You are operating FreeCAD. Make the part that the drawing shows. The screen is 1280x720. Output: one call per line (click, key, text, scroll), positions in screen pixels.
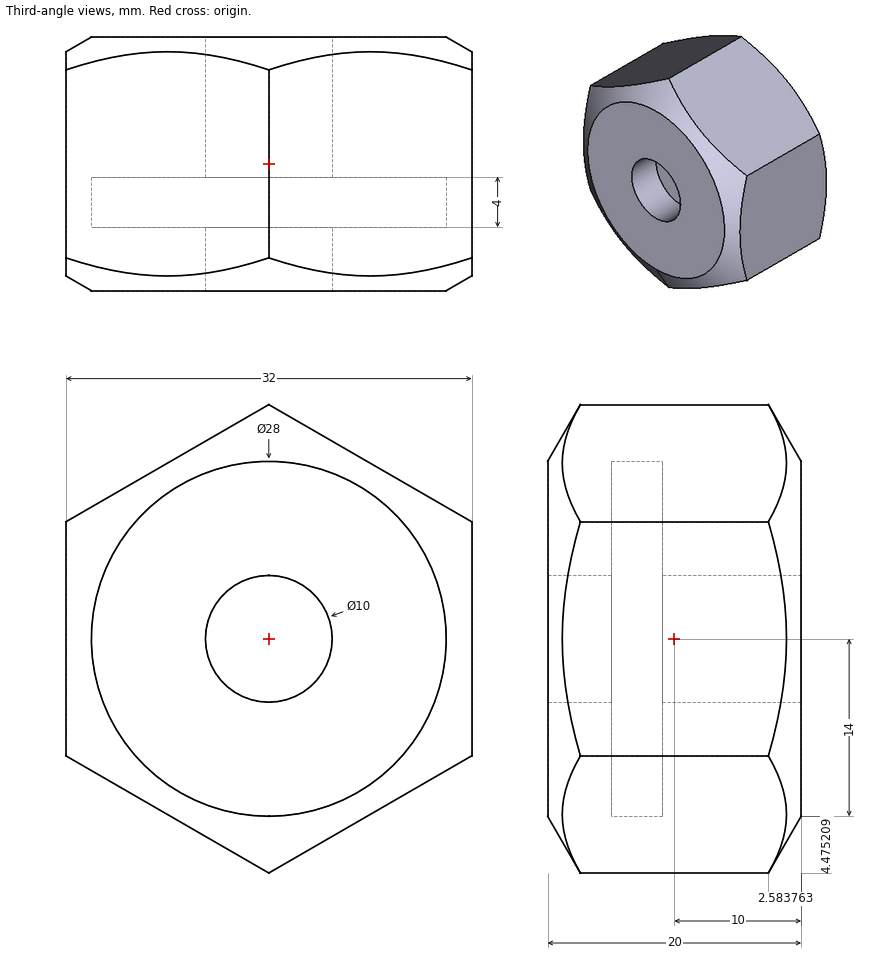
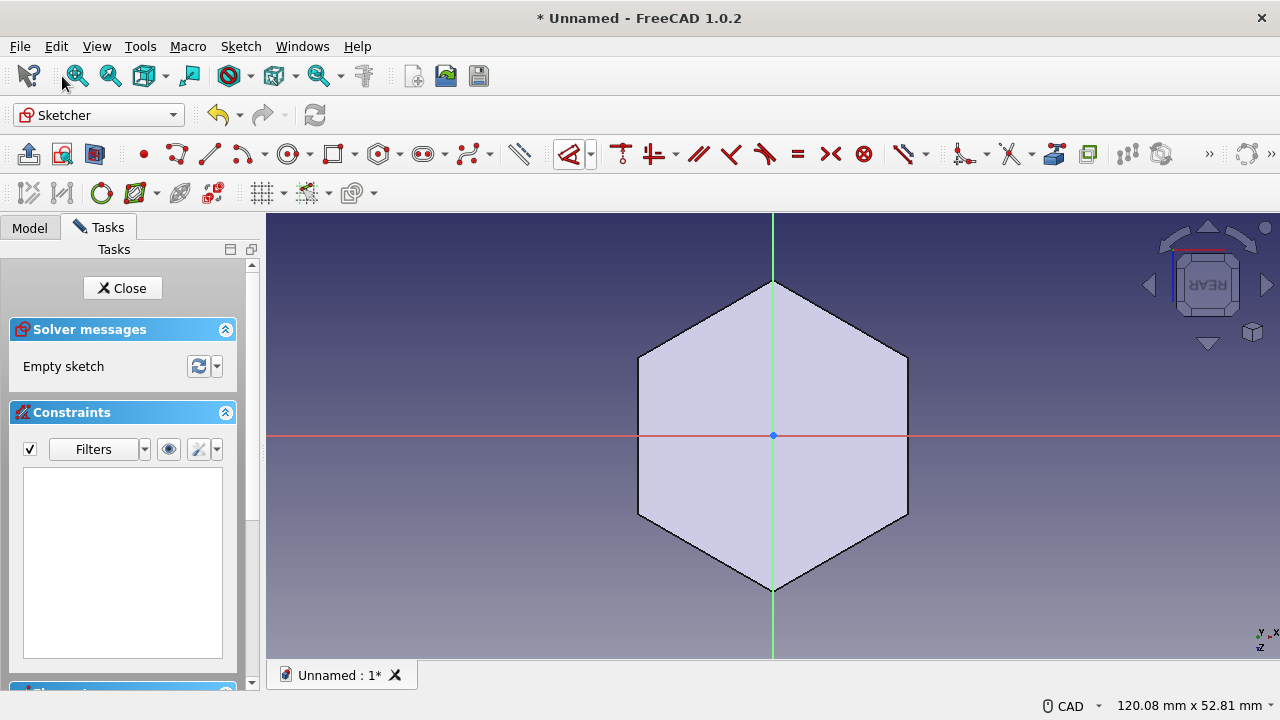
scroll(803, 436, up, 6)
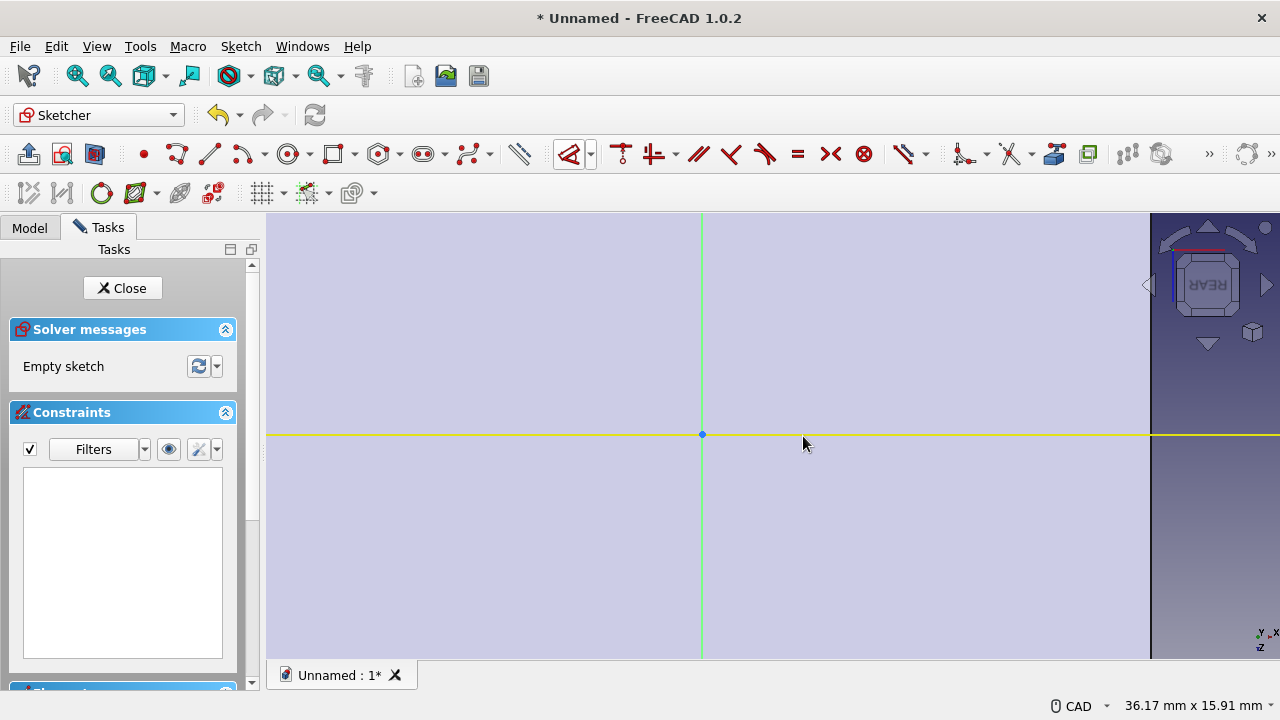
click(288, 154)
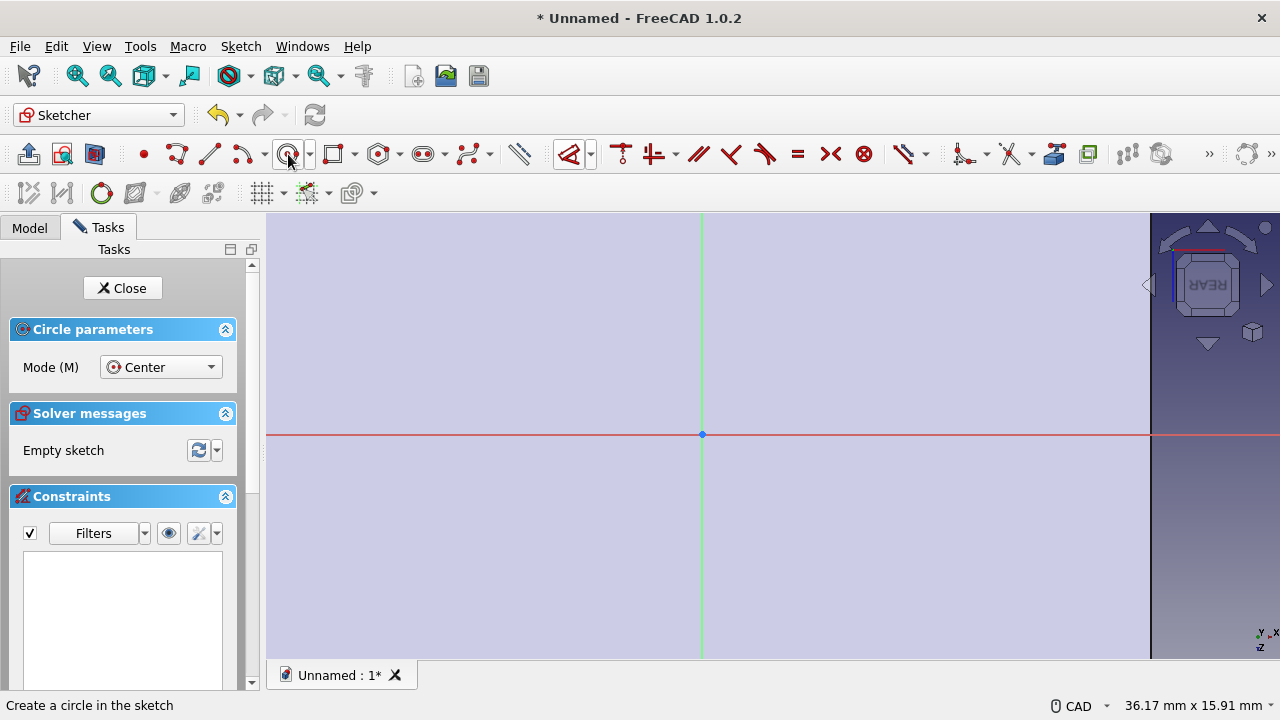
click(702, 435)
click(801, 336)
key(Escape)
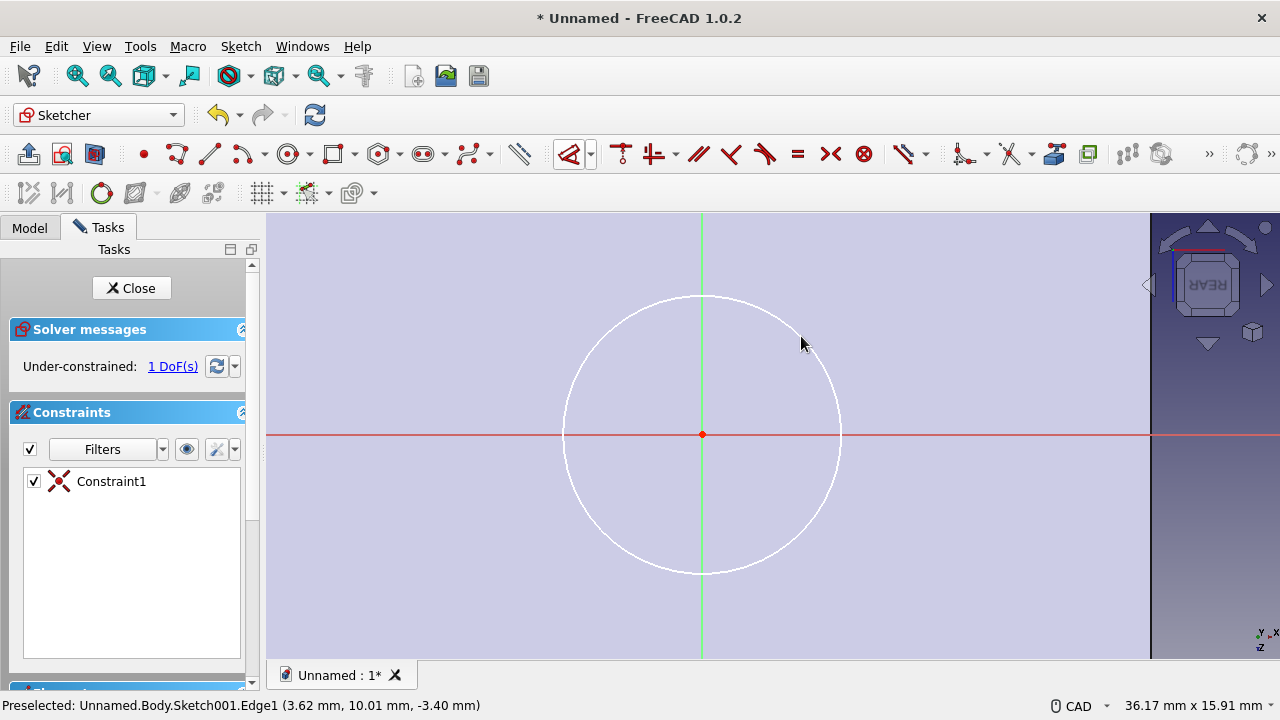
click(800, 336)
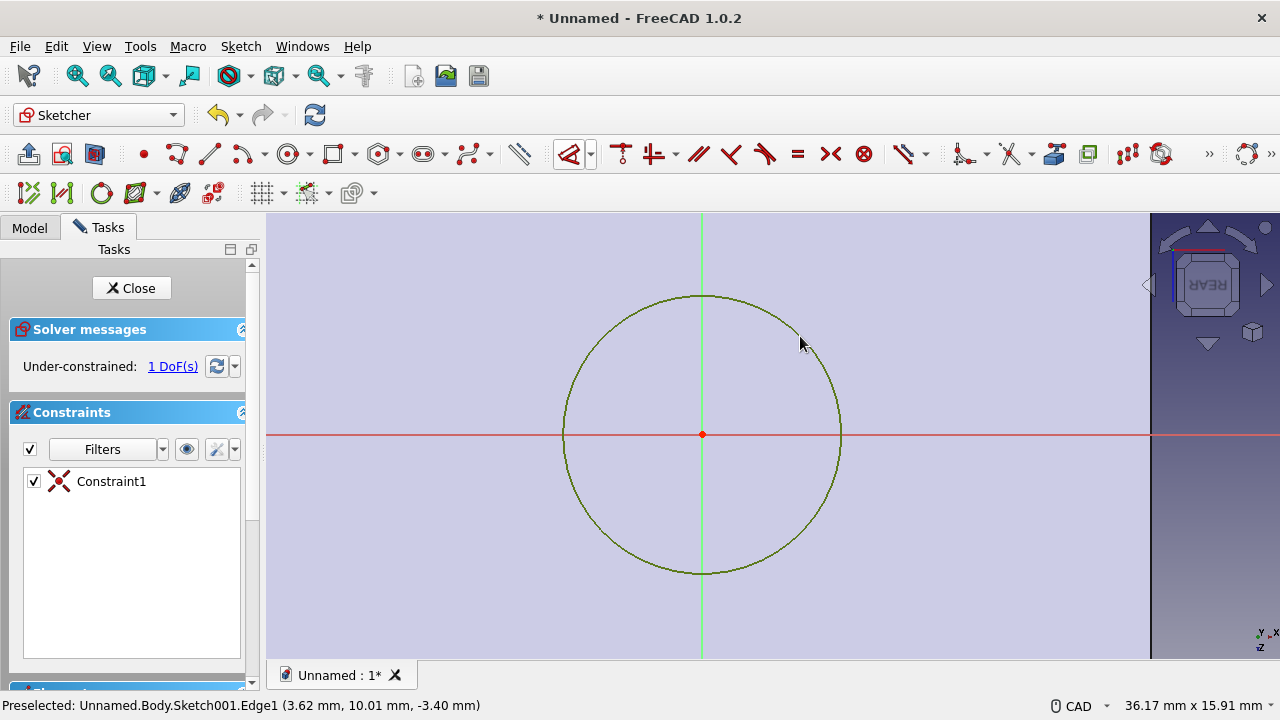
key(k)
key(o)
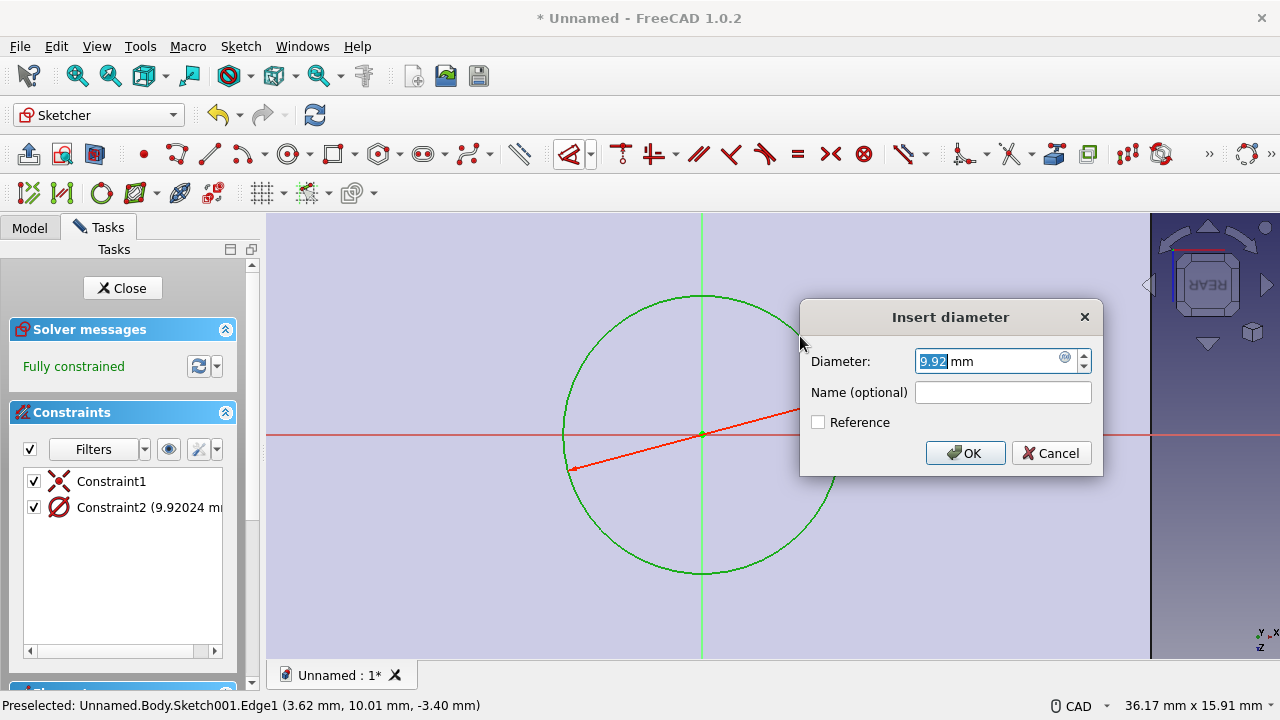
text(10)
key(Return)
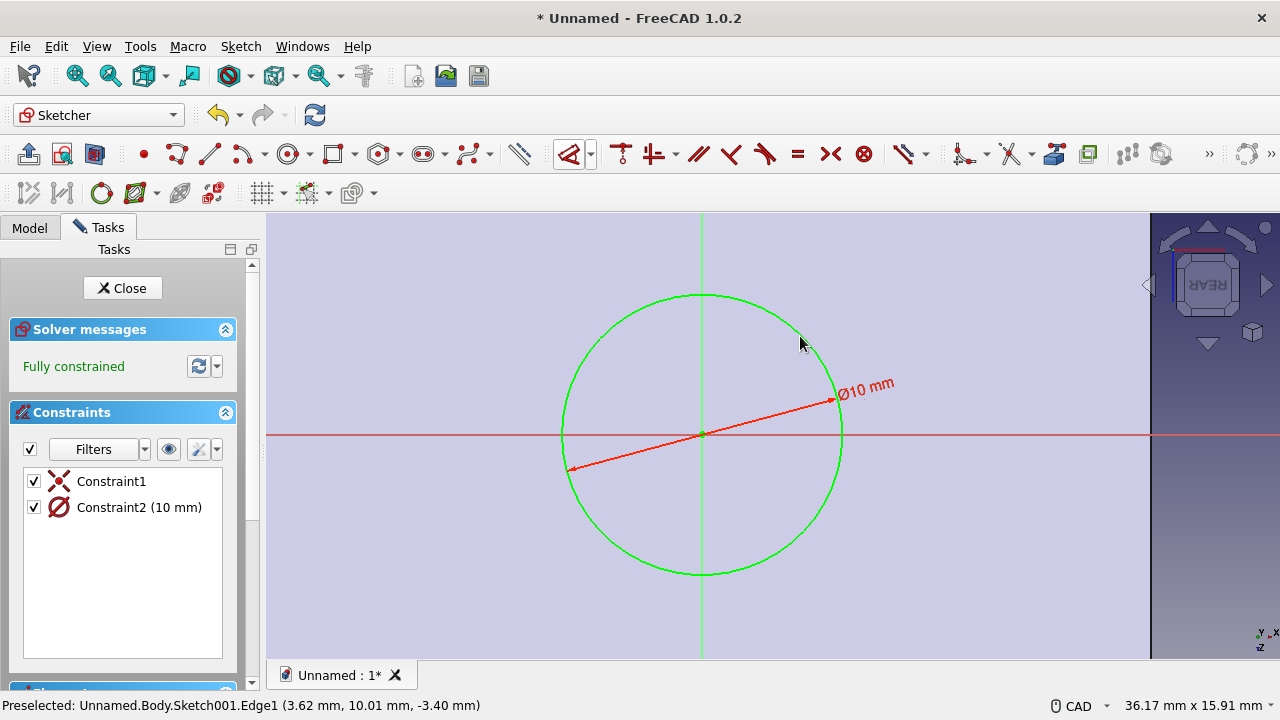
click(123, 288)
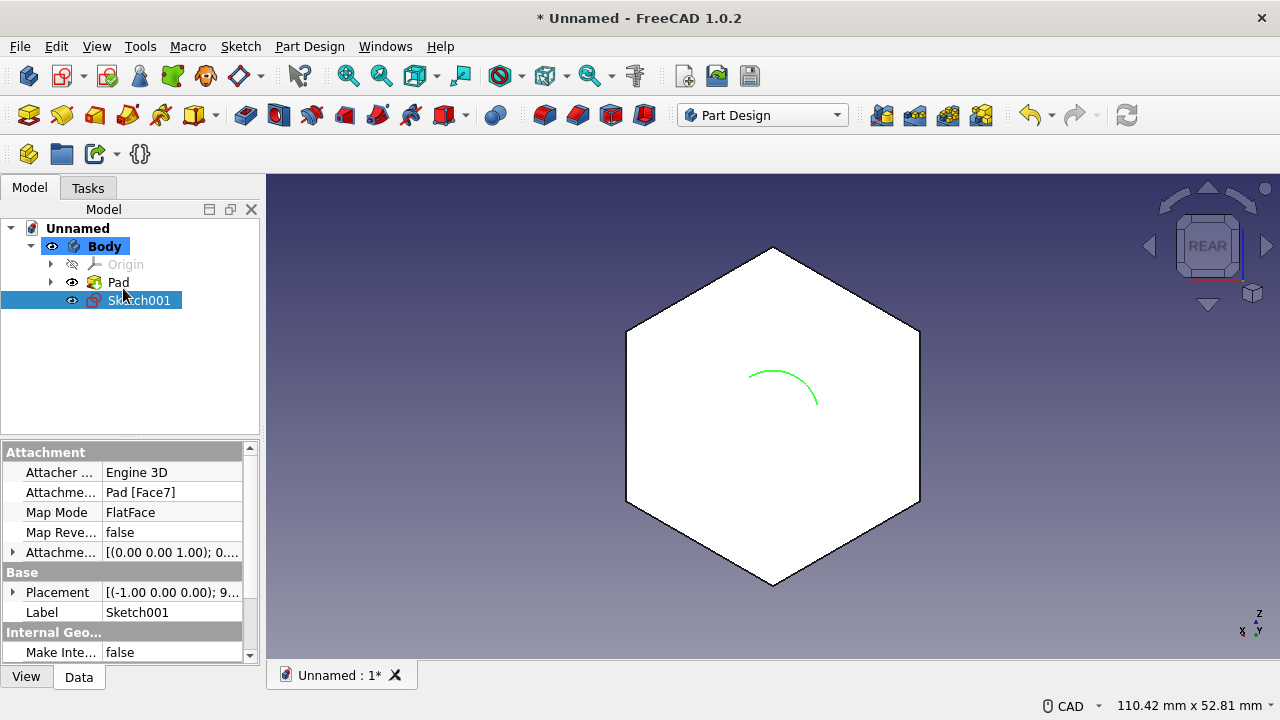
click(246, 116)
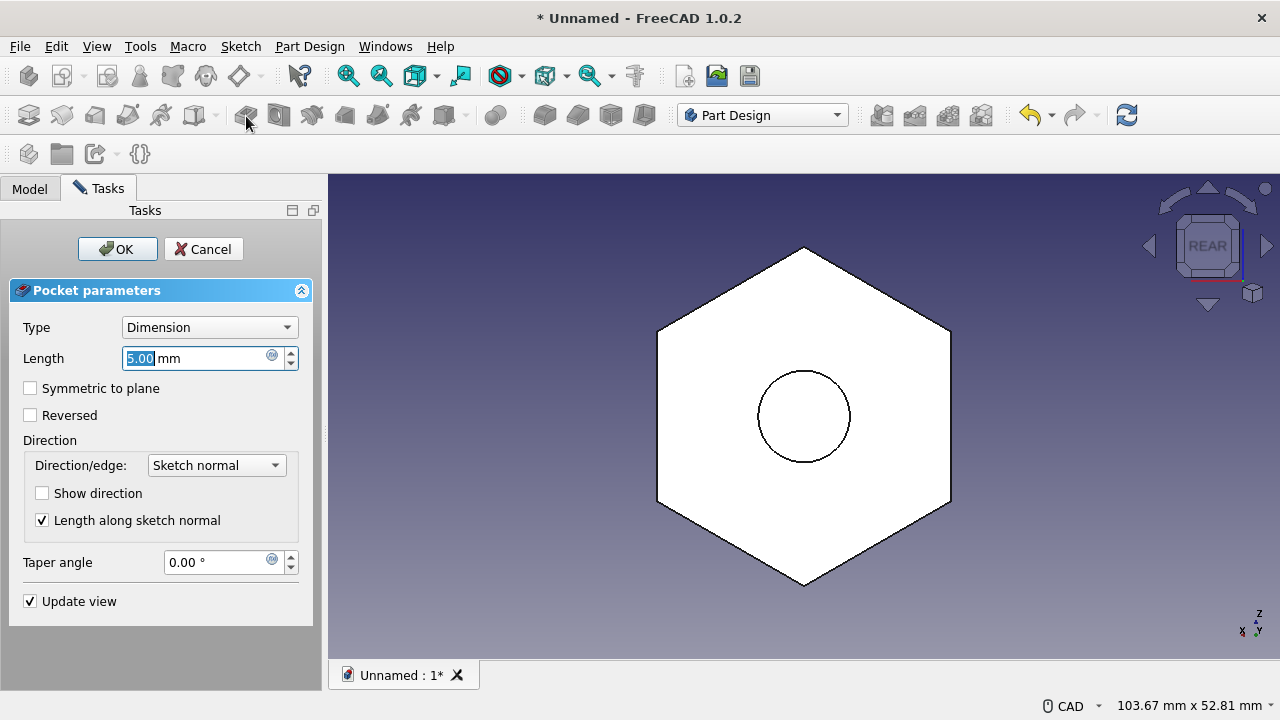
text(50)
key(Tab)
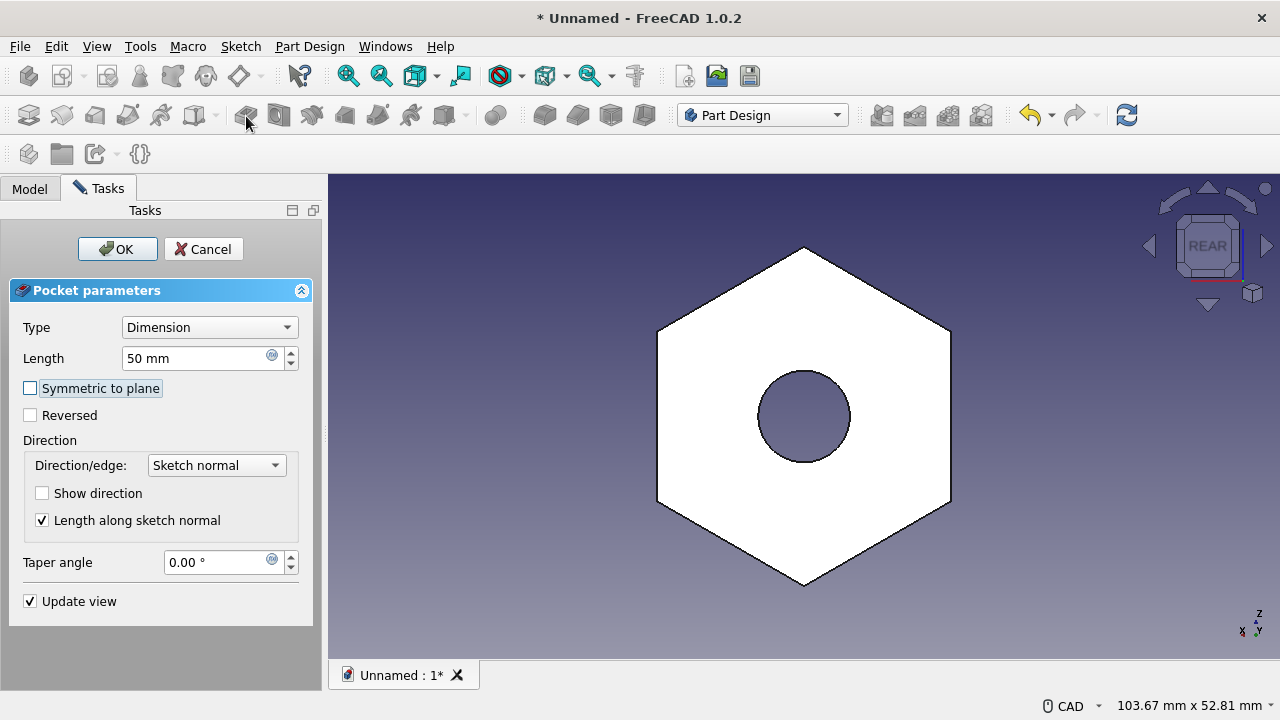
click(118, 249)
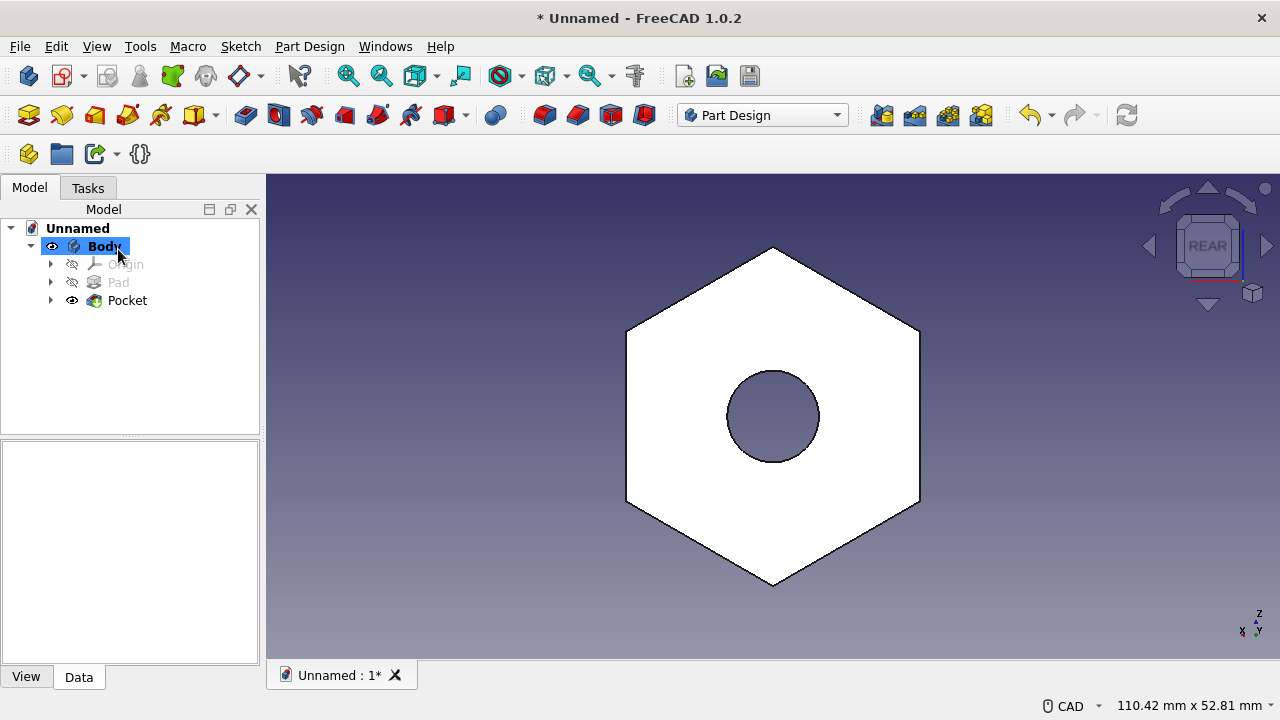
click(51, 264)